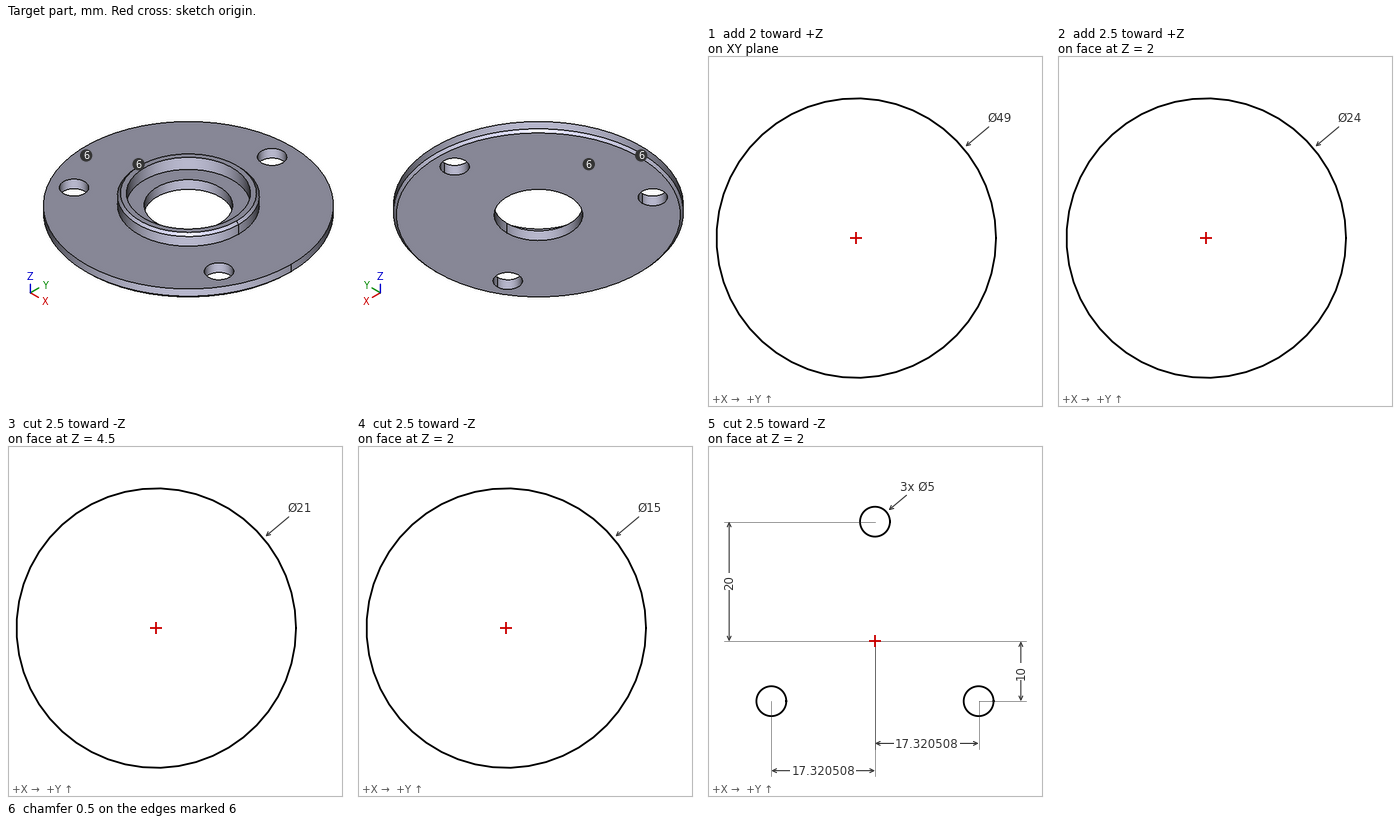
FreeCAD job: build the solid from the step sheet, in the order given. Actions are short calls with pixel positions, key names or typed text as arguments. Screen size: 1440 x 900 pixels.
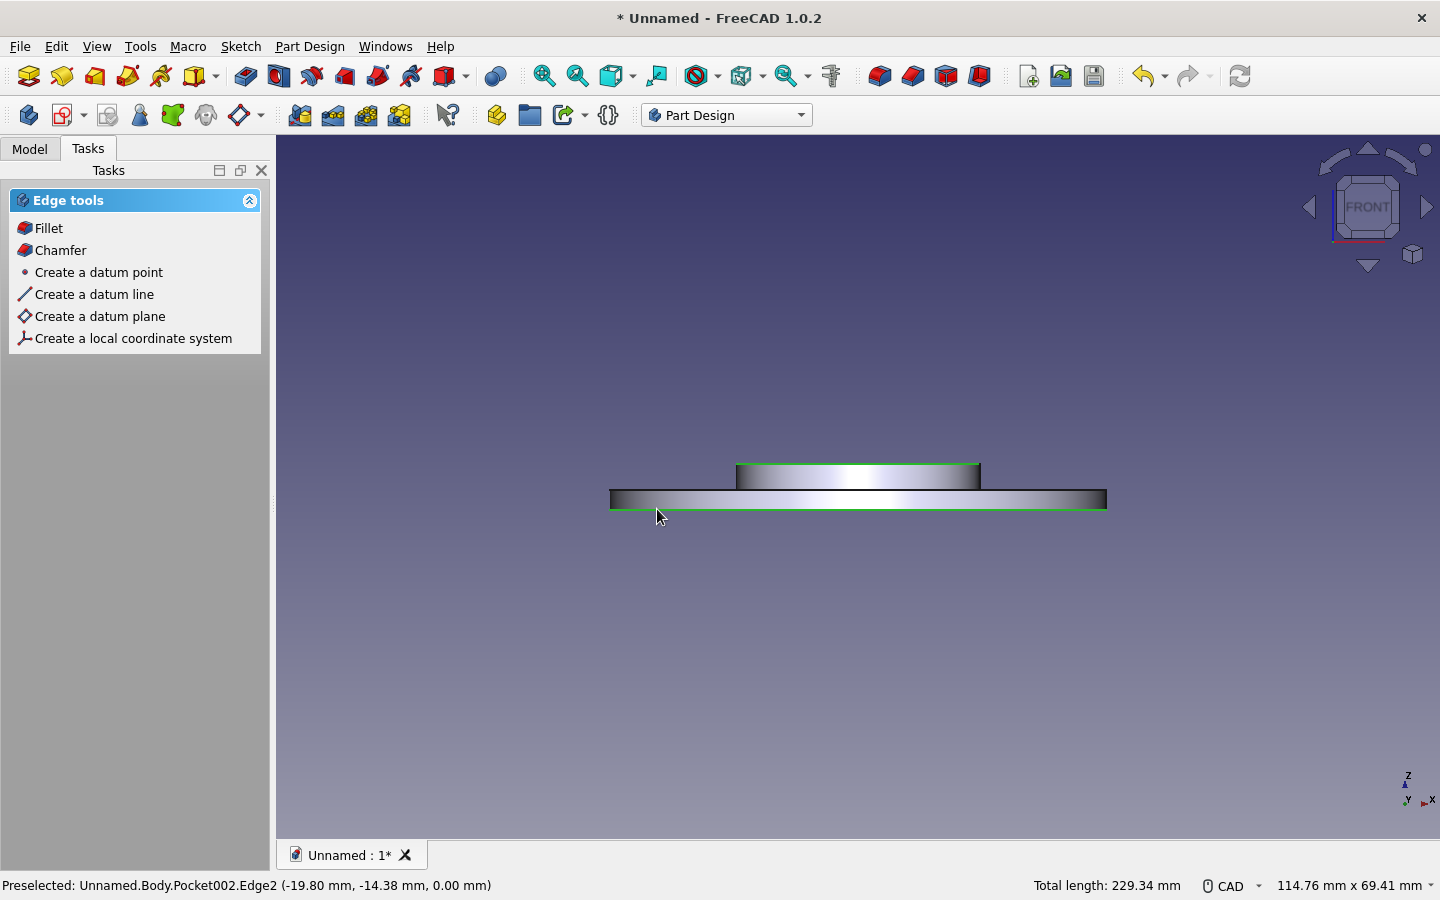
click(913, 76)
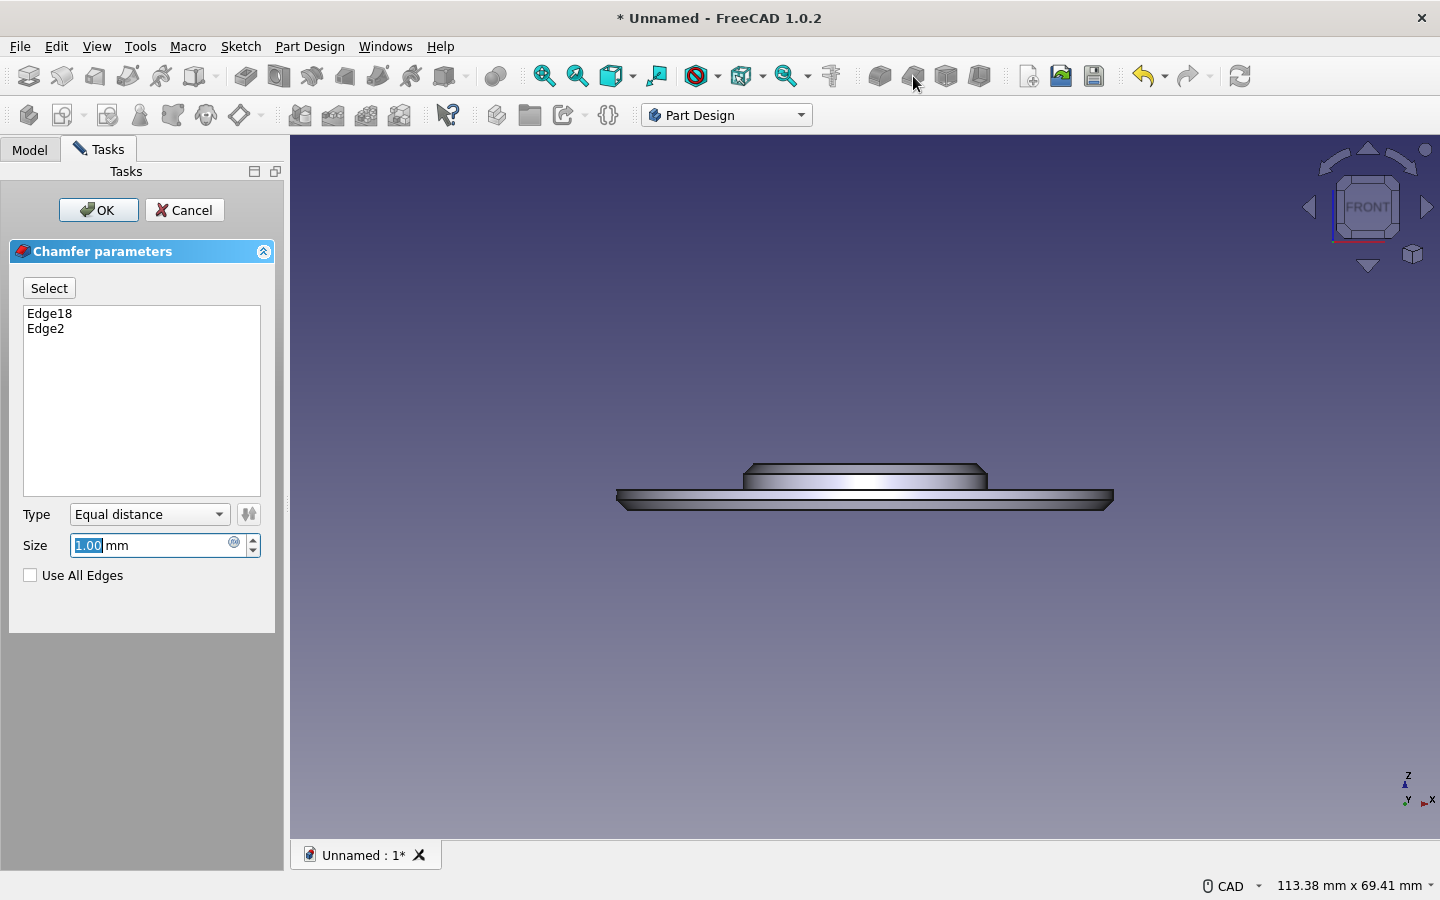
text(0.5)
key(Tab)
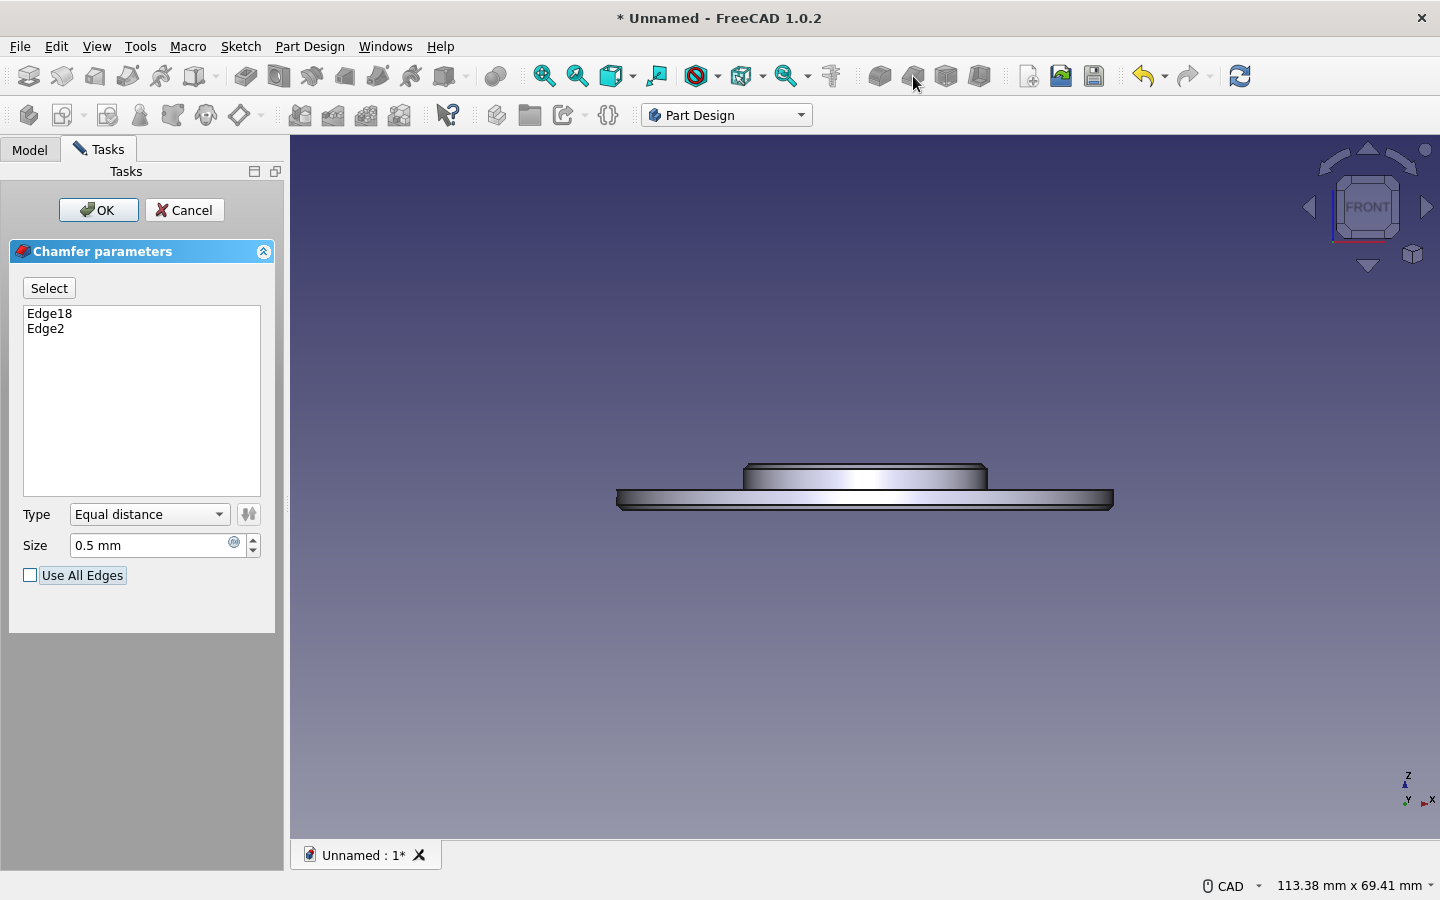
click(99, 210)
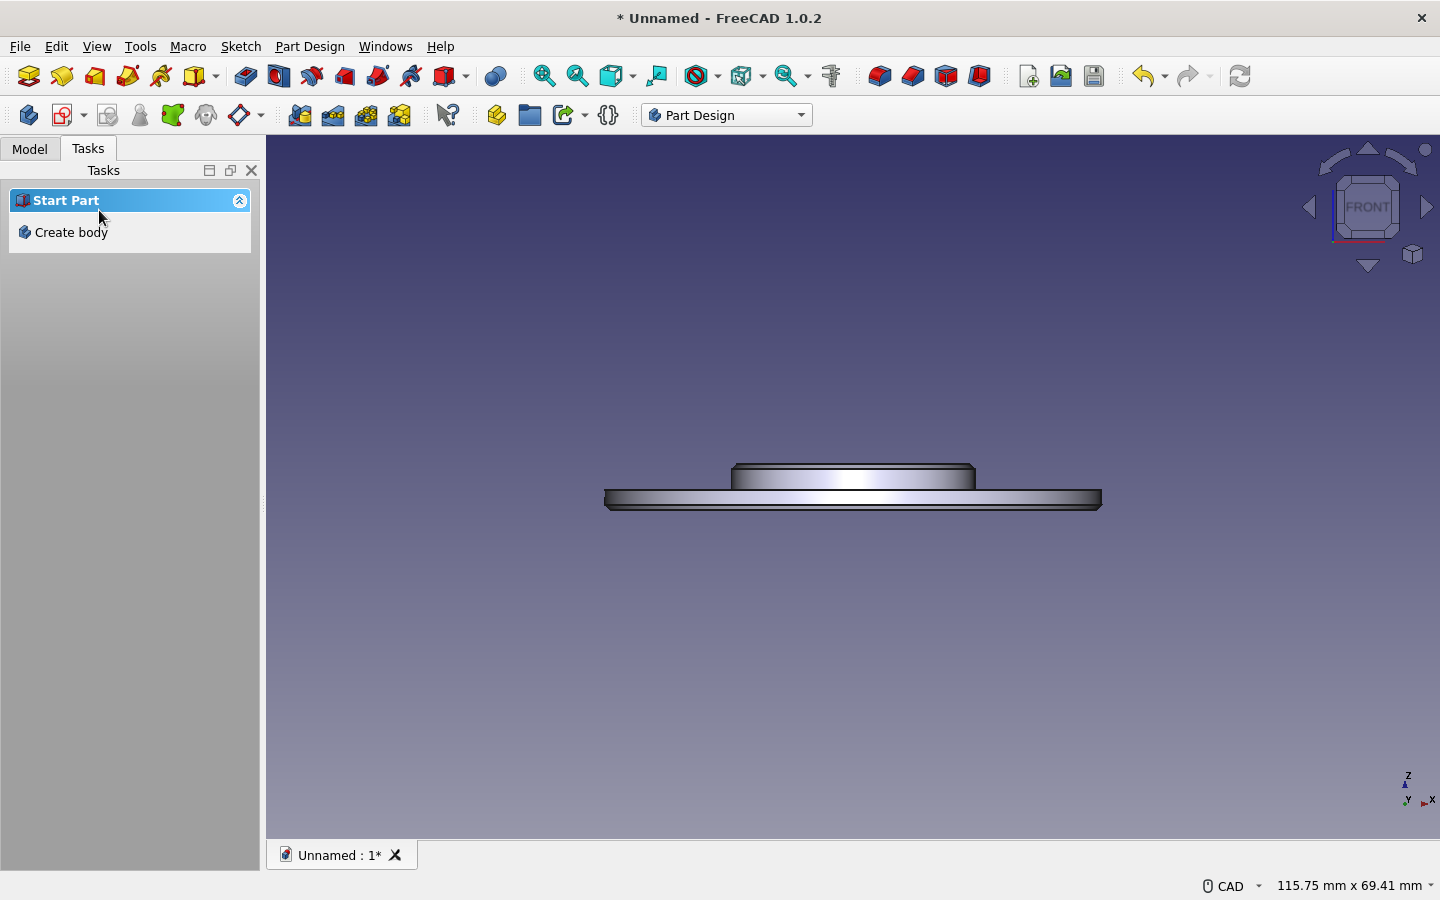
key(0)